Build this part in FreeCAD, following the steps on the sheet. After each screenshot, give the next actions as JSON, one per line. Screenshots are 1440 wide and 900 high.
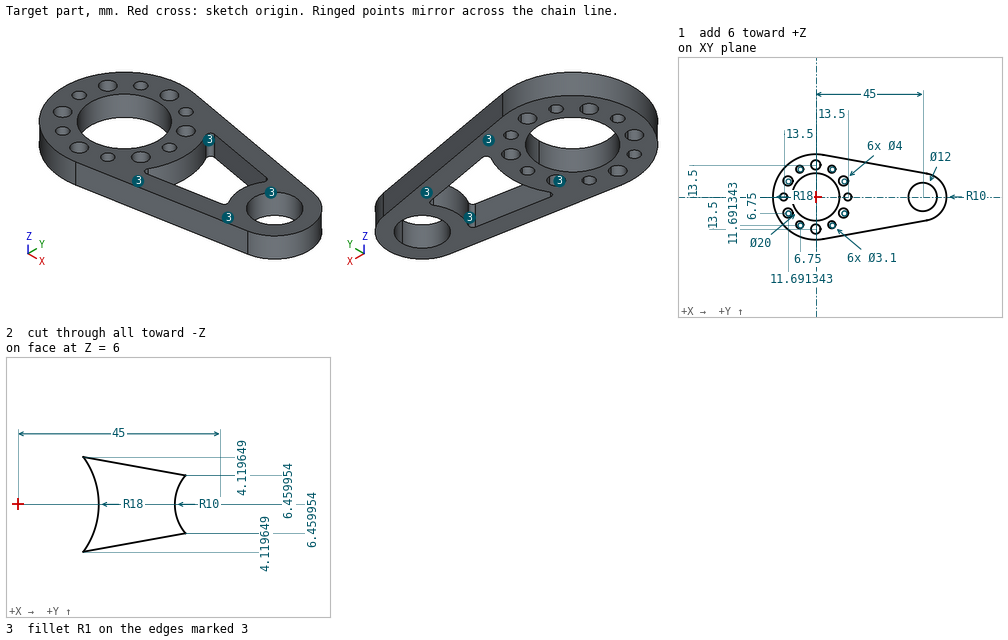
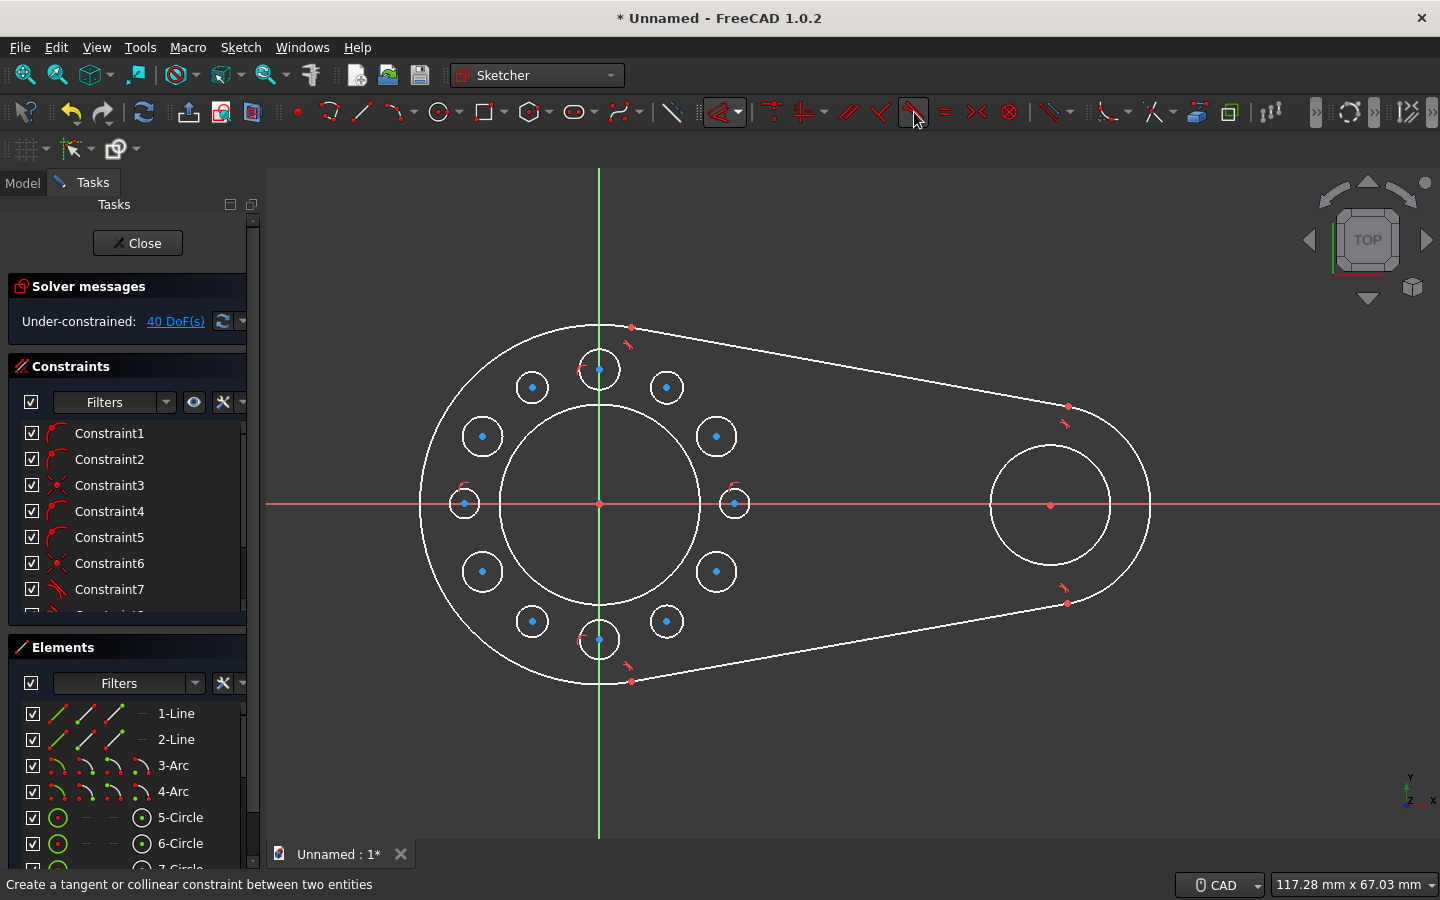
{"action": "scroll", "coordinate": [600, 504], "scroll_direction": "up", "scroll_amount": 5}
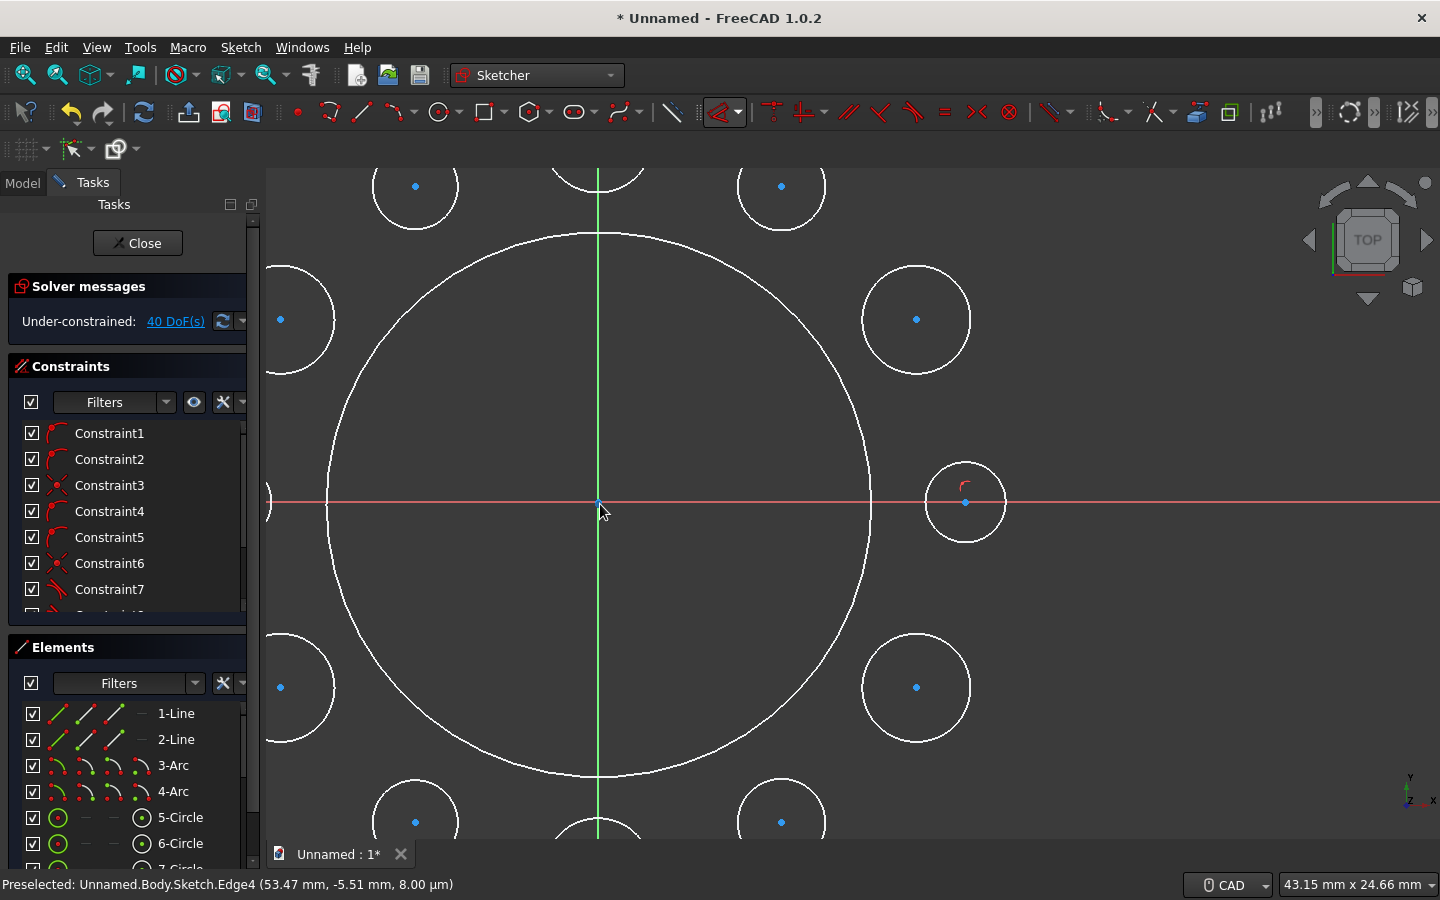
{"action": "left_click_drag", "start_coordinate": [588, 492], "coordinate": [609, 515]}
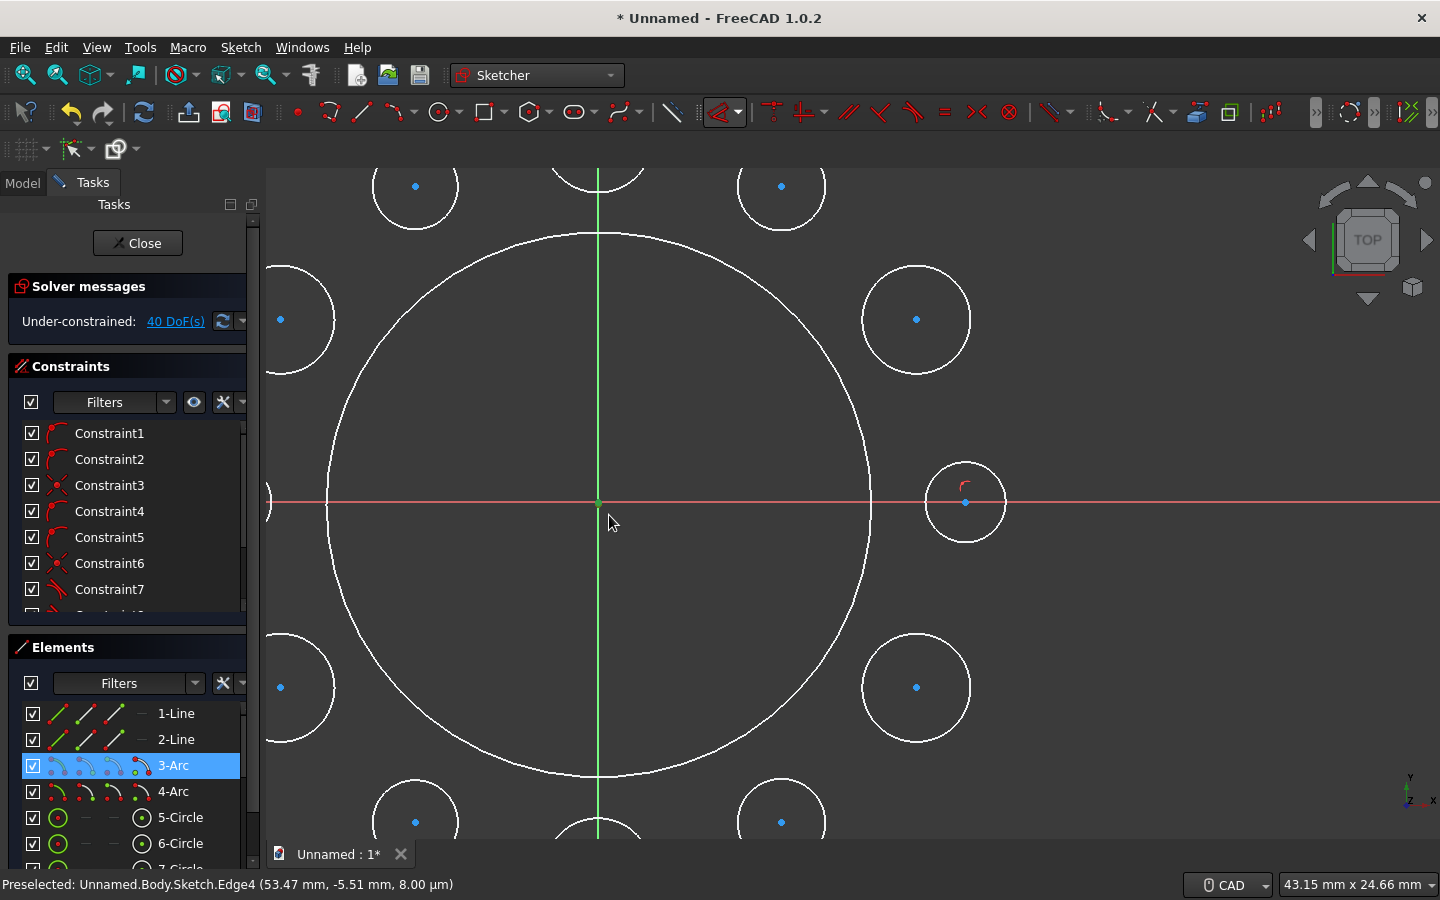
{"action": "key", "text": "c"}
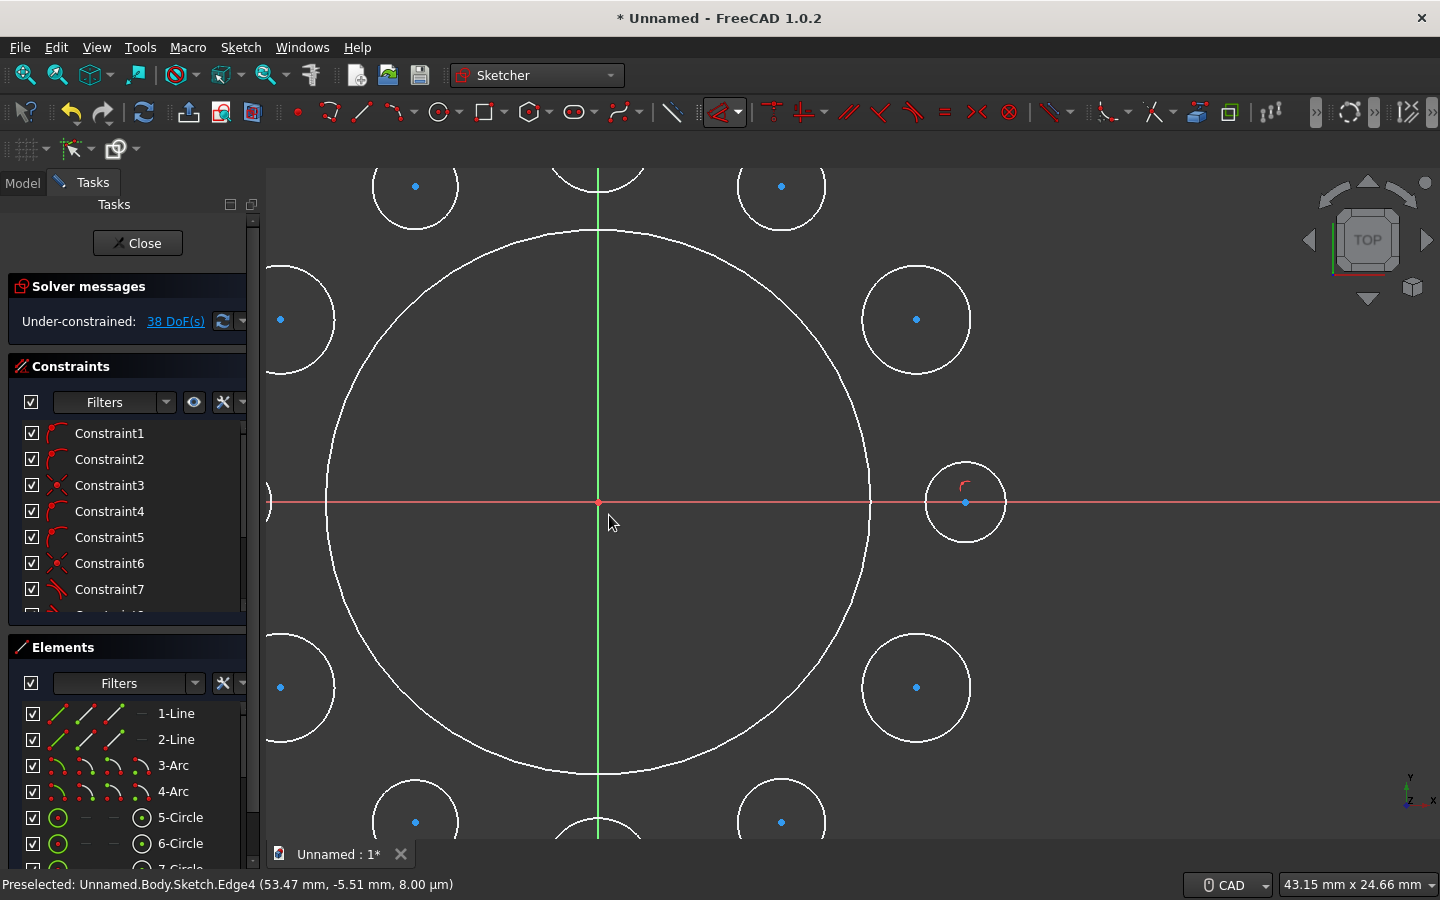
{"action": "left_click", "coordinate": [445, 793]}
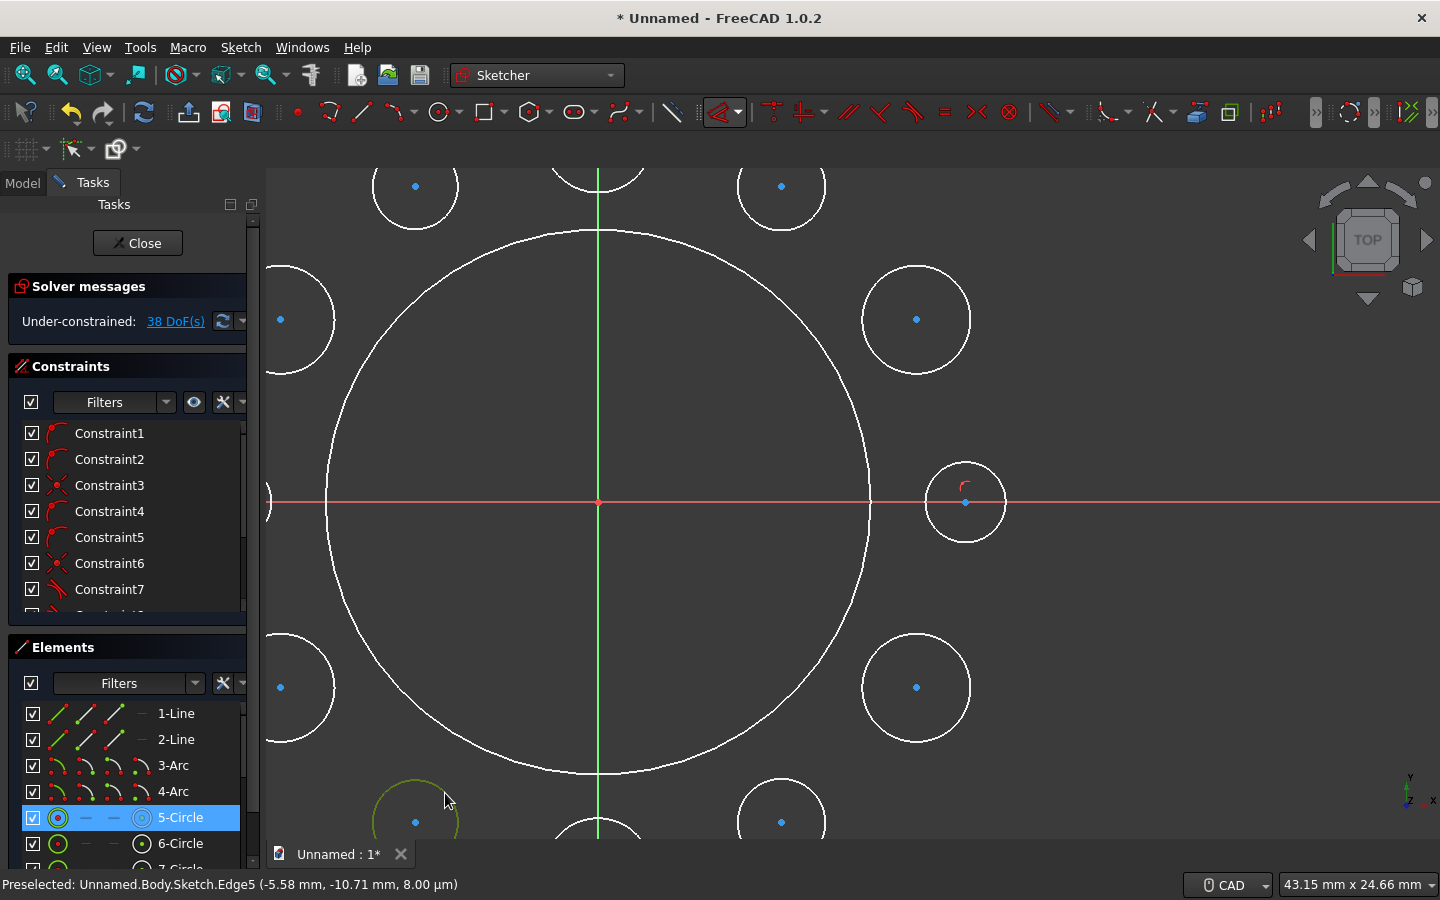
{"action": "left_click", "coordinate": [812, 792]}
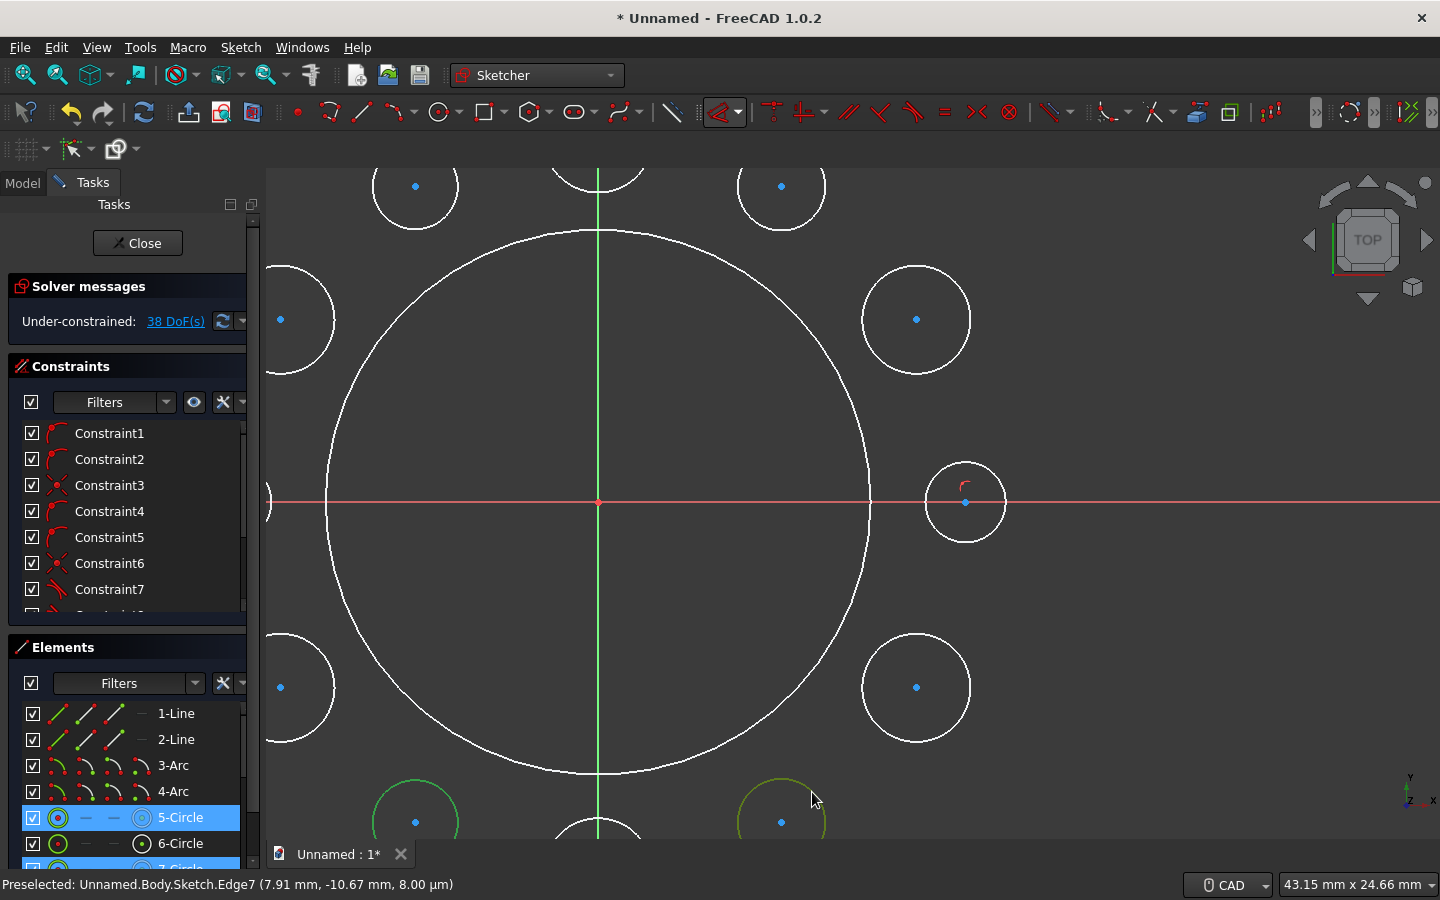
{"action": "scroll", "coordinate": [600, 504], "scroll_direction": "down", "scroll_amount": 5}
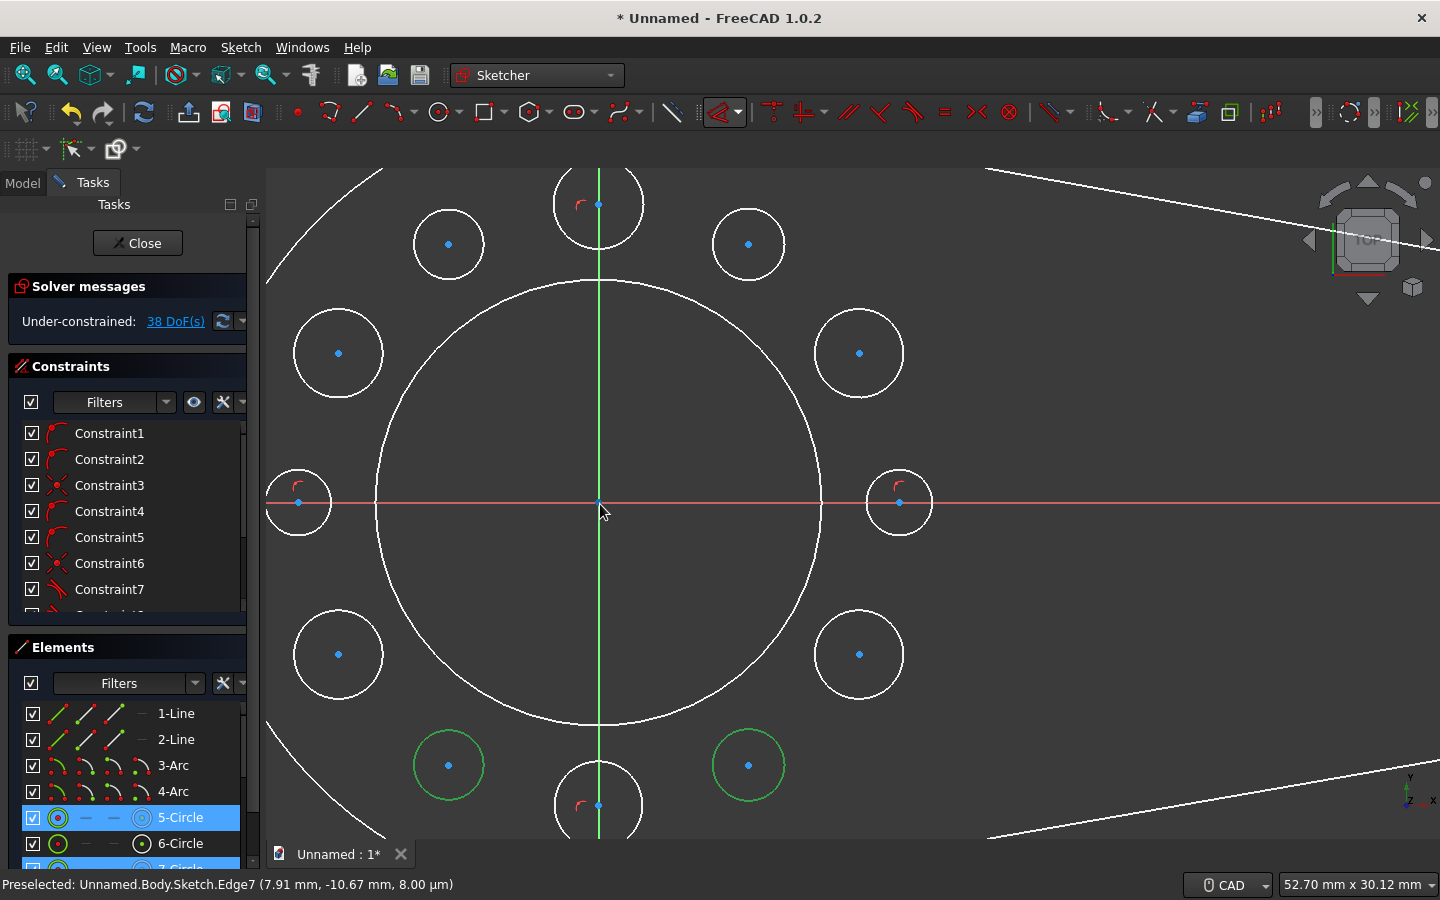
{"action": "scroll", "coordinate": [475, 493], "scroll_direction": "up", "scroll_amount": 2}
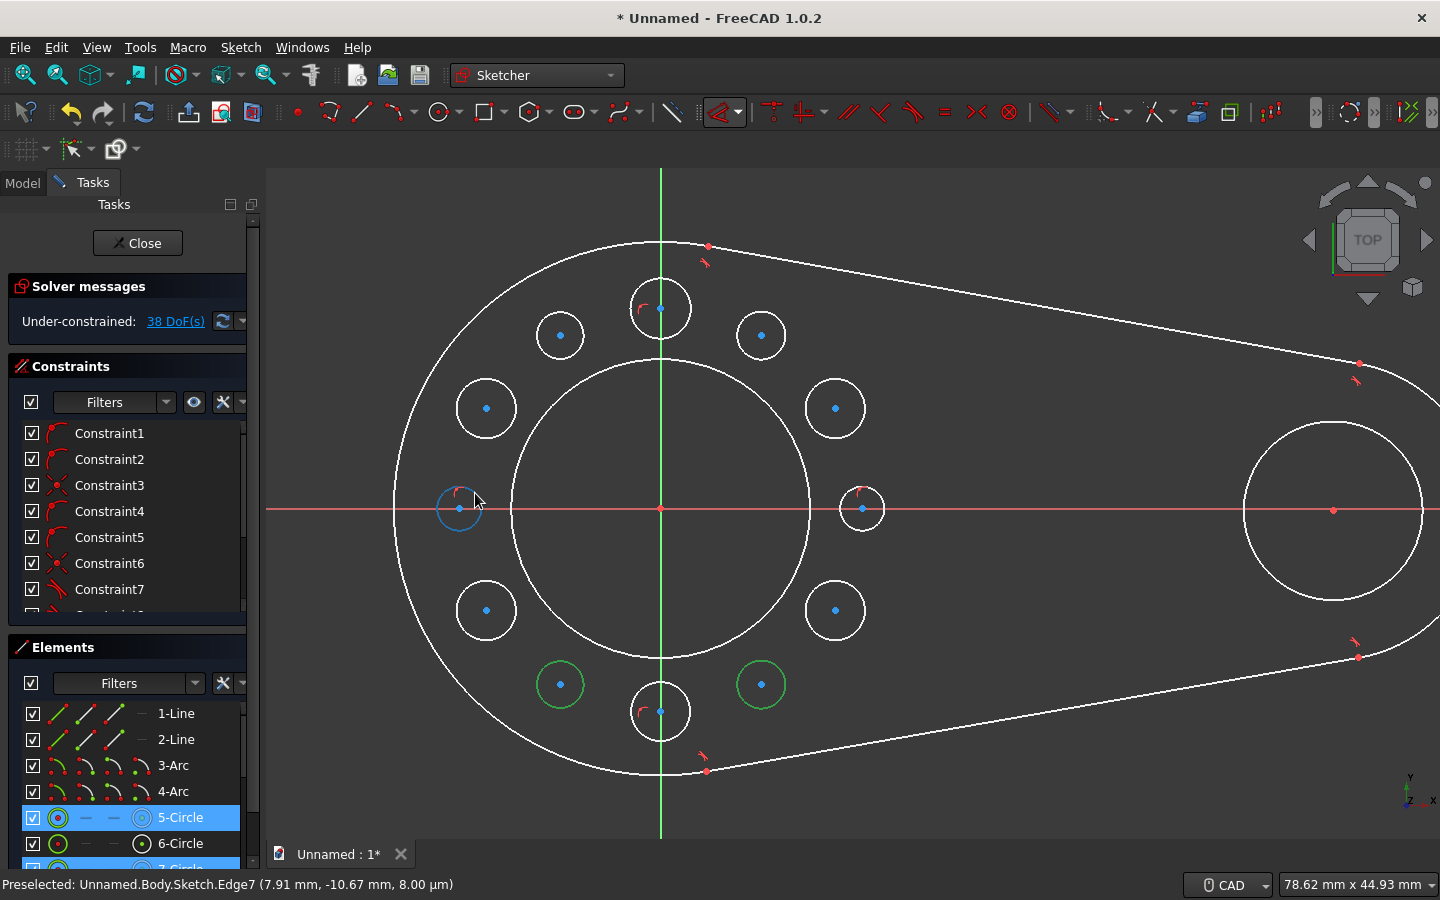
{"action": "left_click", "coordinate": [475, 493]}